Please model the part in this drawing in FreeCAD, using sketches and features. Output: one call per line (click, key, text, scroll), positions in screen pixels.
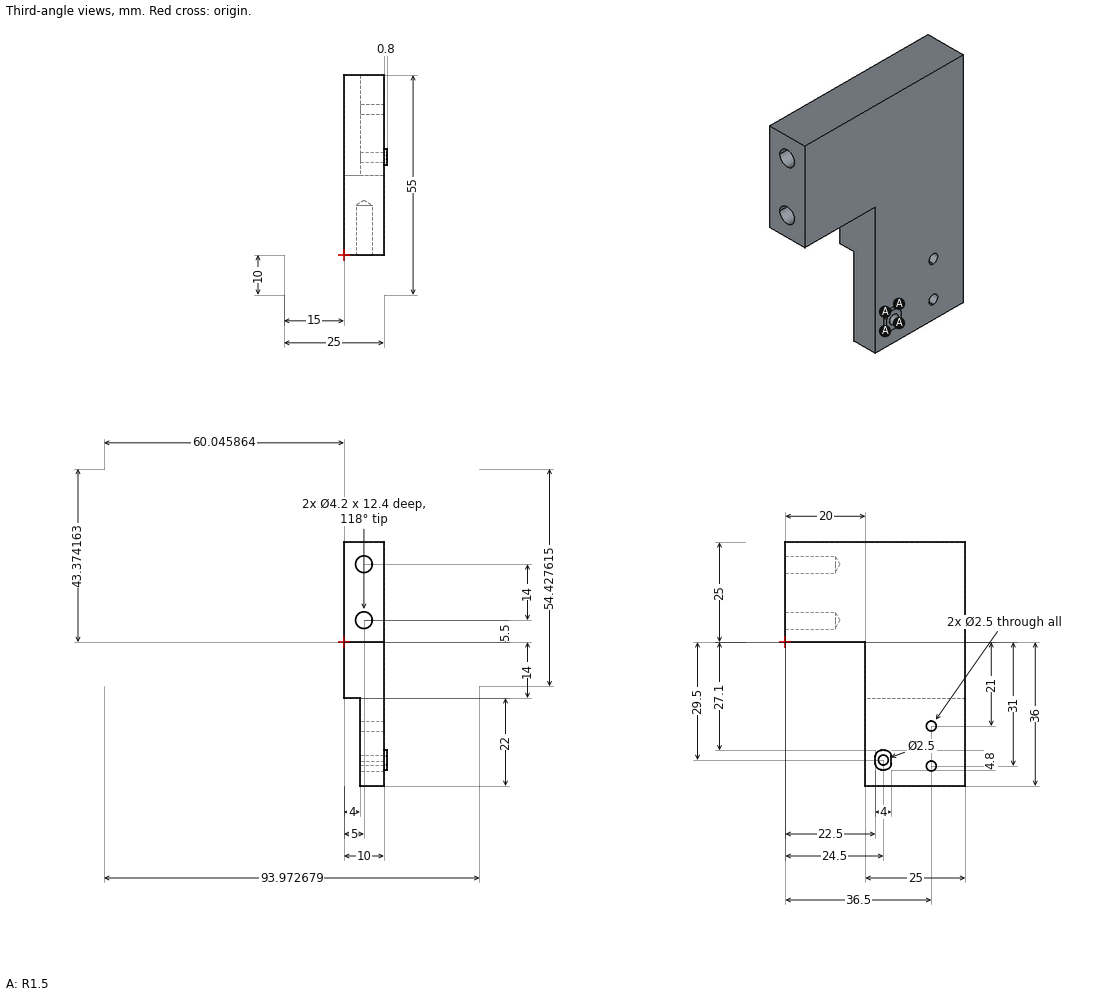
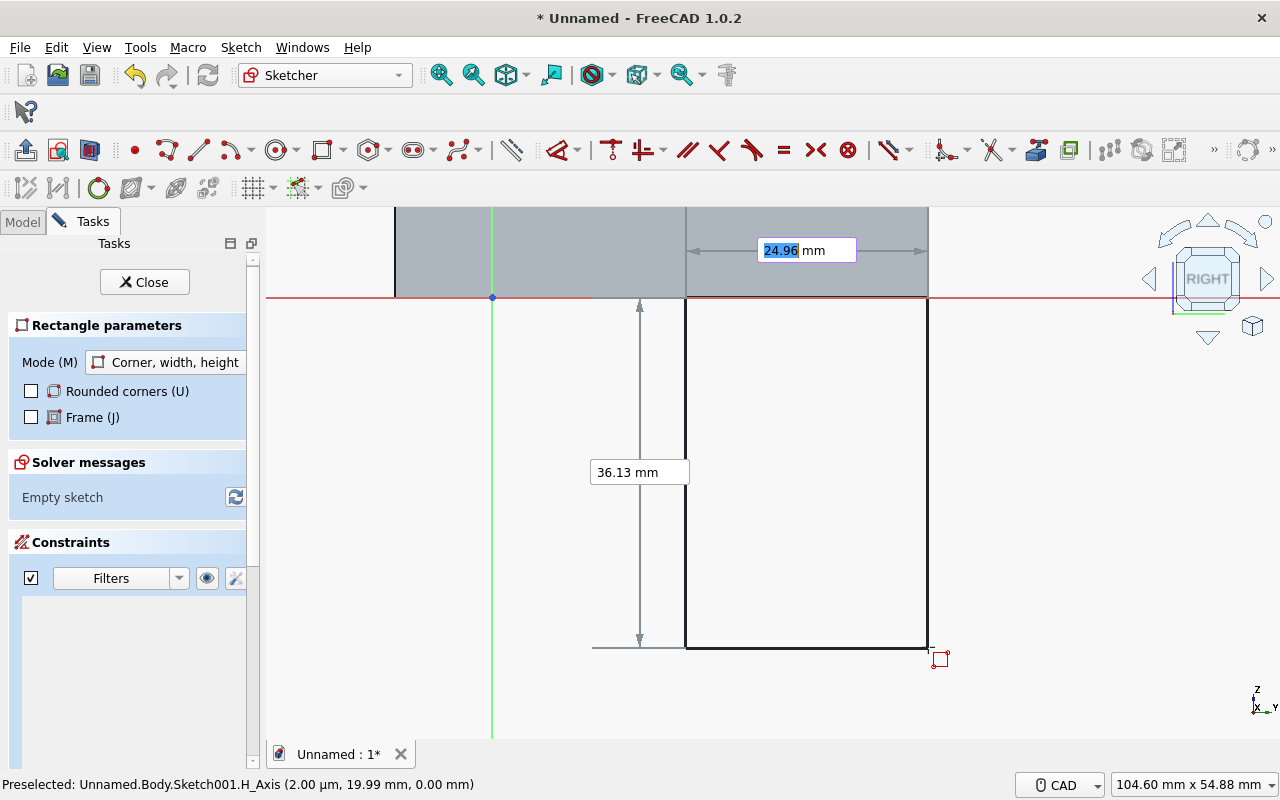
text(25)
key(Tab)
text(36)
key(Return)
key(Escape)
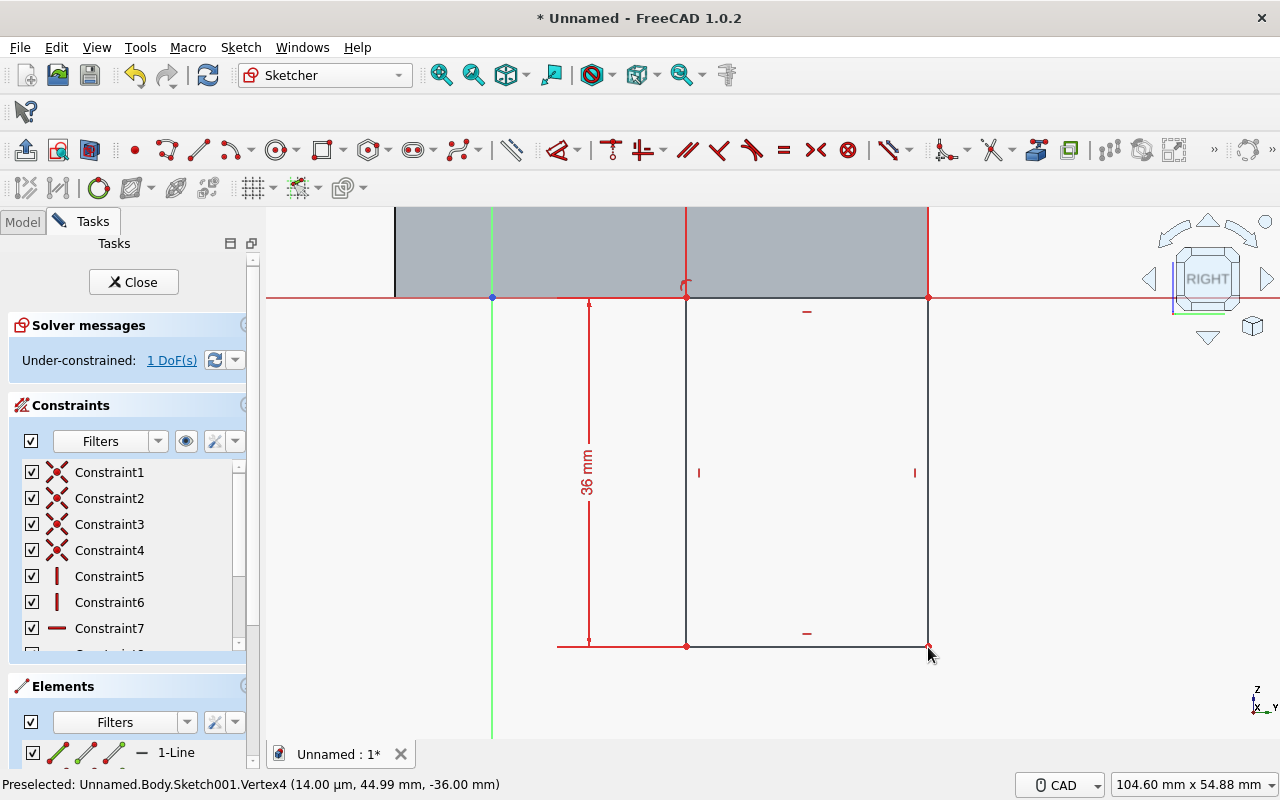
key(d)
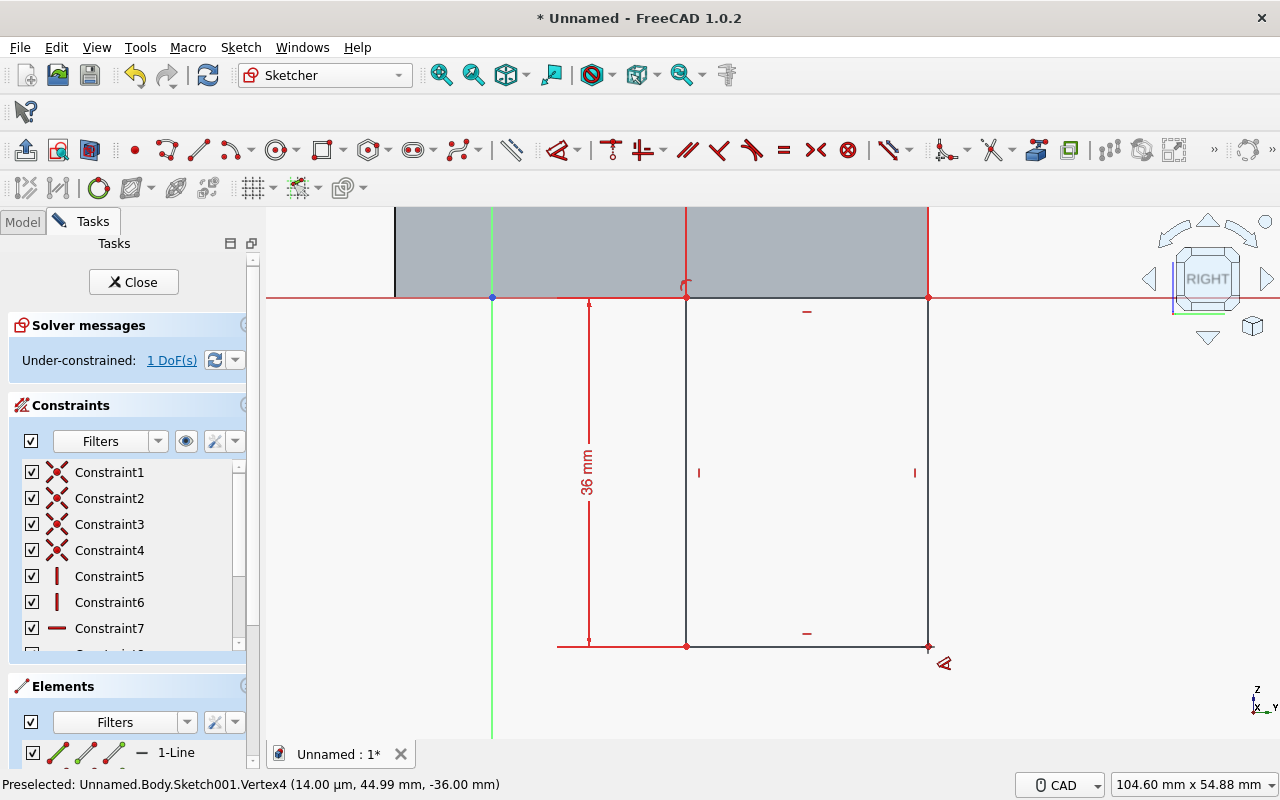
click(686, 298)
click(589, 264)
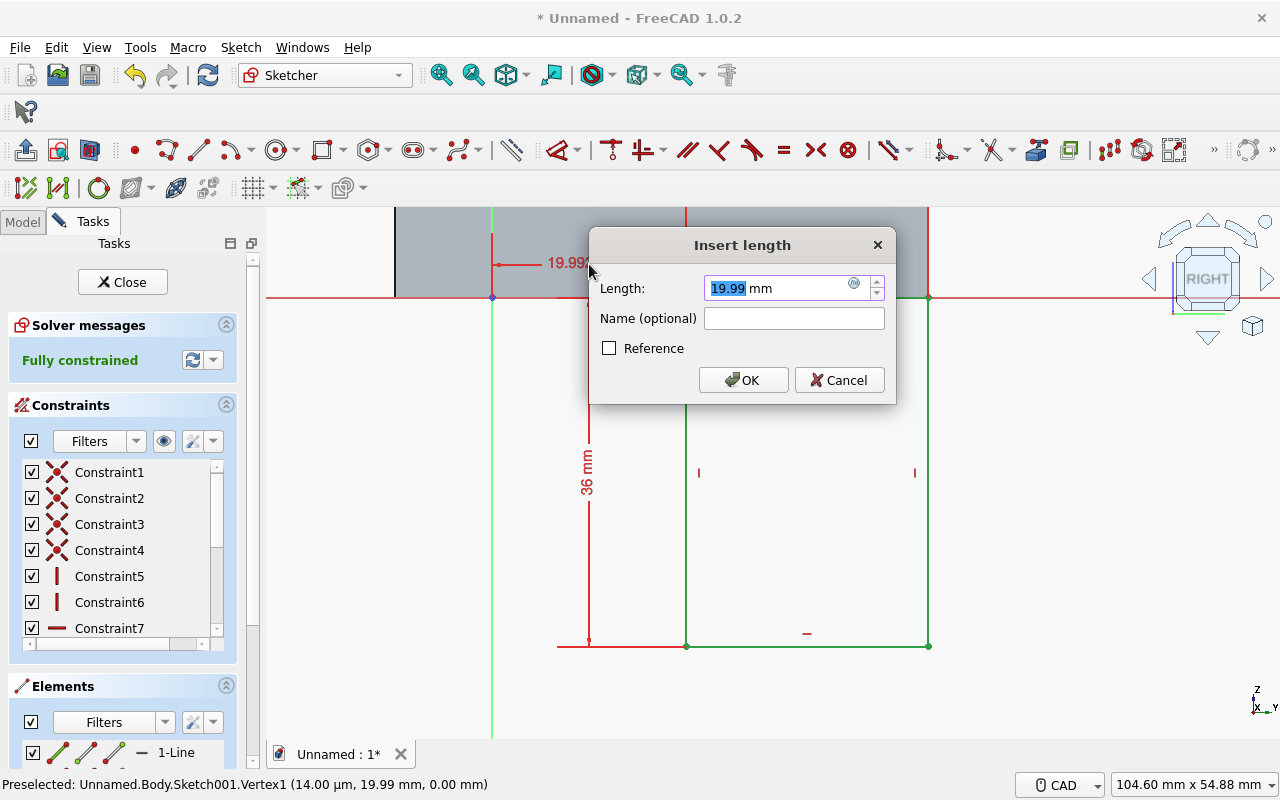
text(20)
key(Return)
key(Escape)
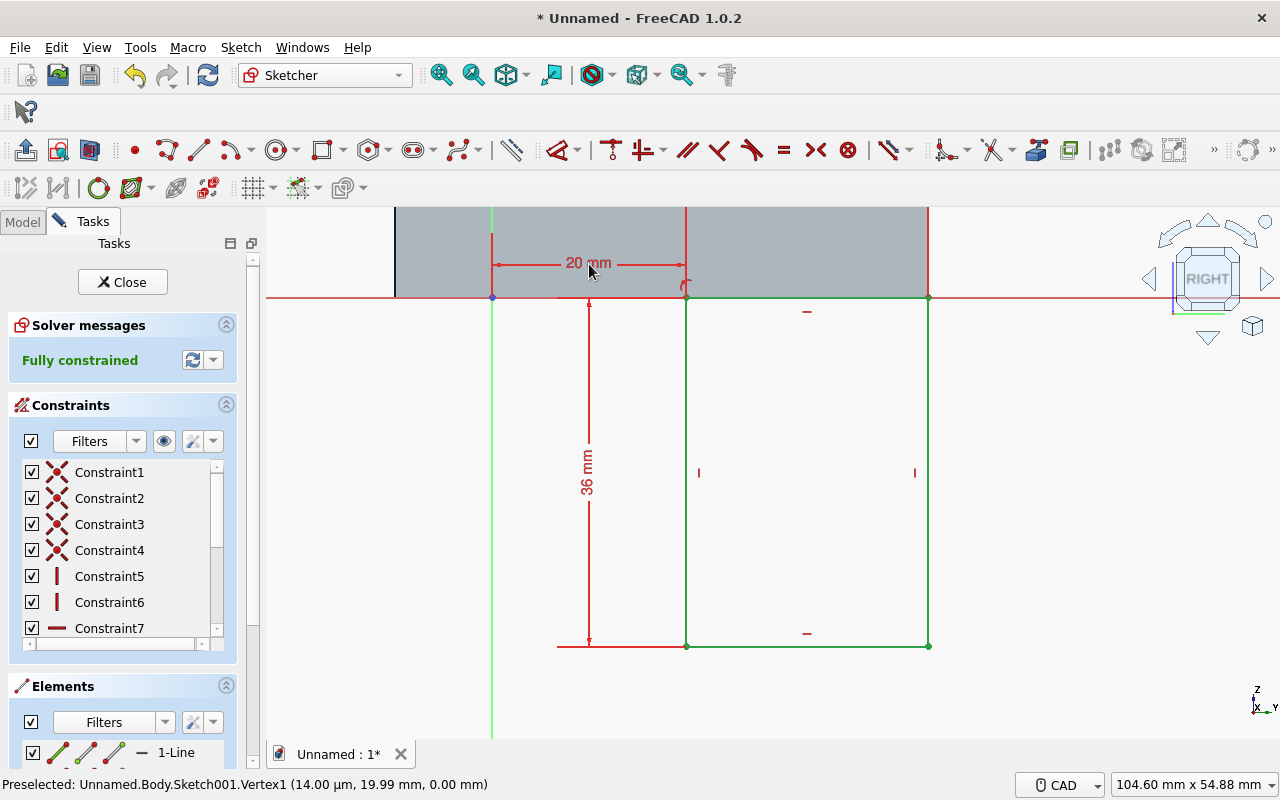
click(123, 282)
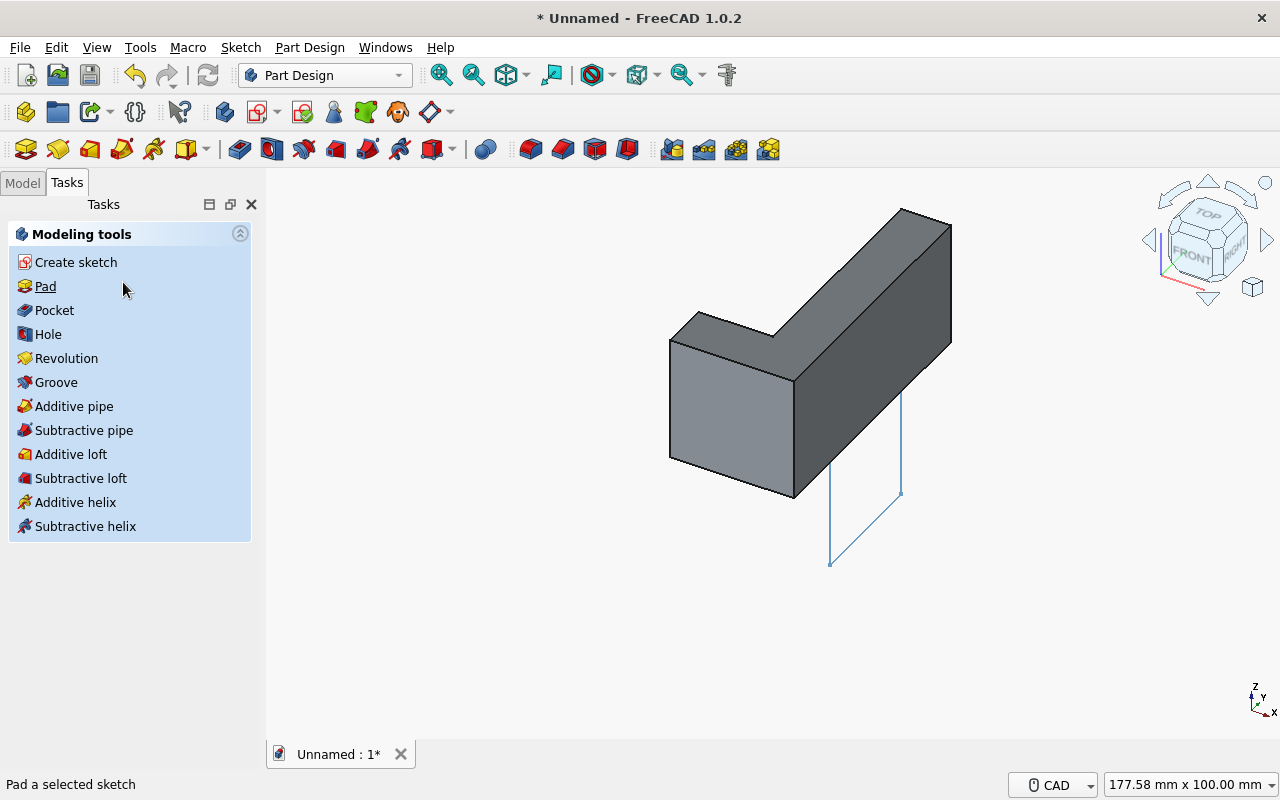
click(26, 150)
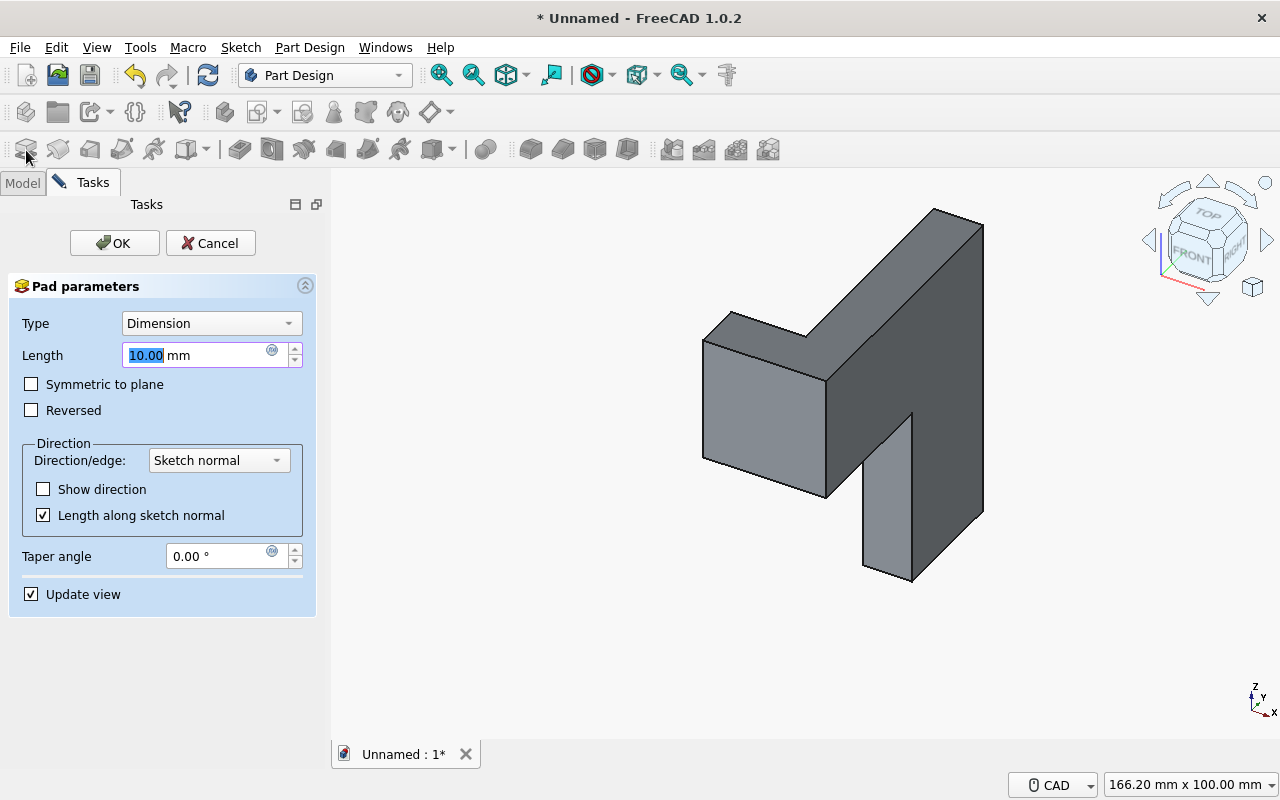
text(10)
key(Tab)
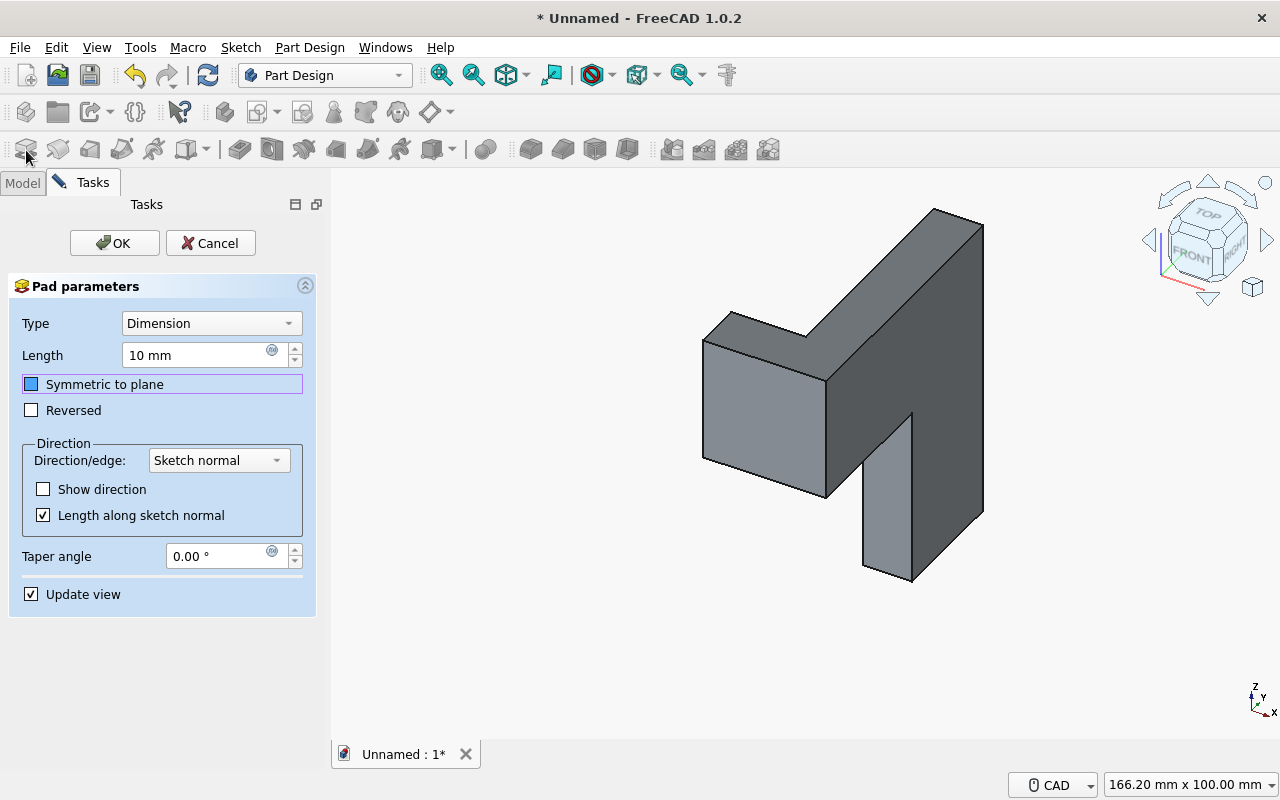
click(115, 243)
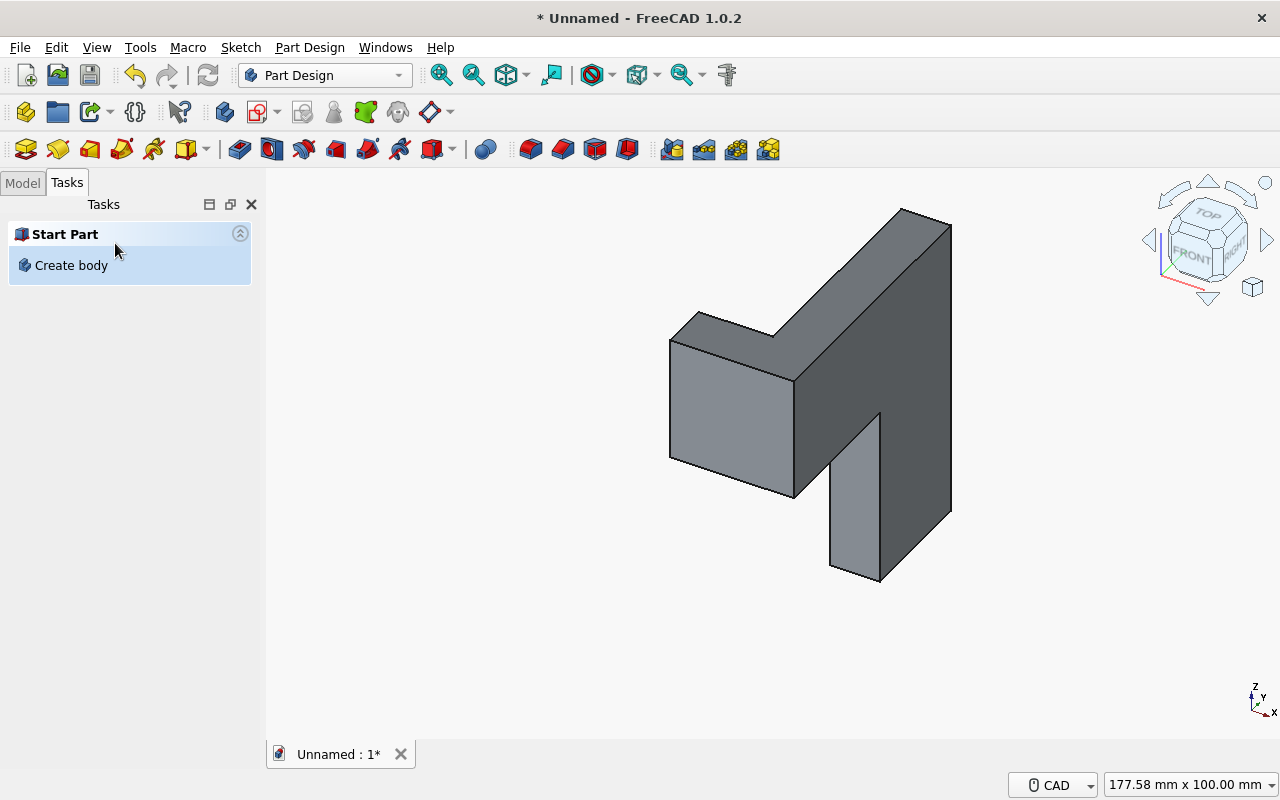
key(4)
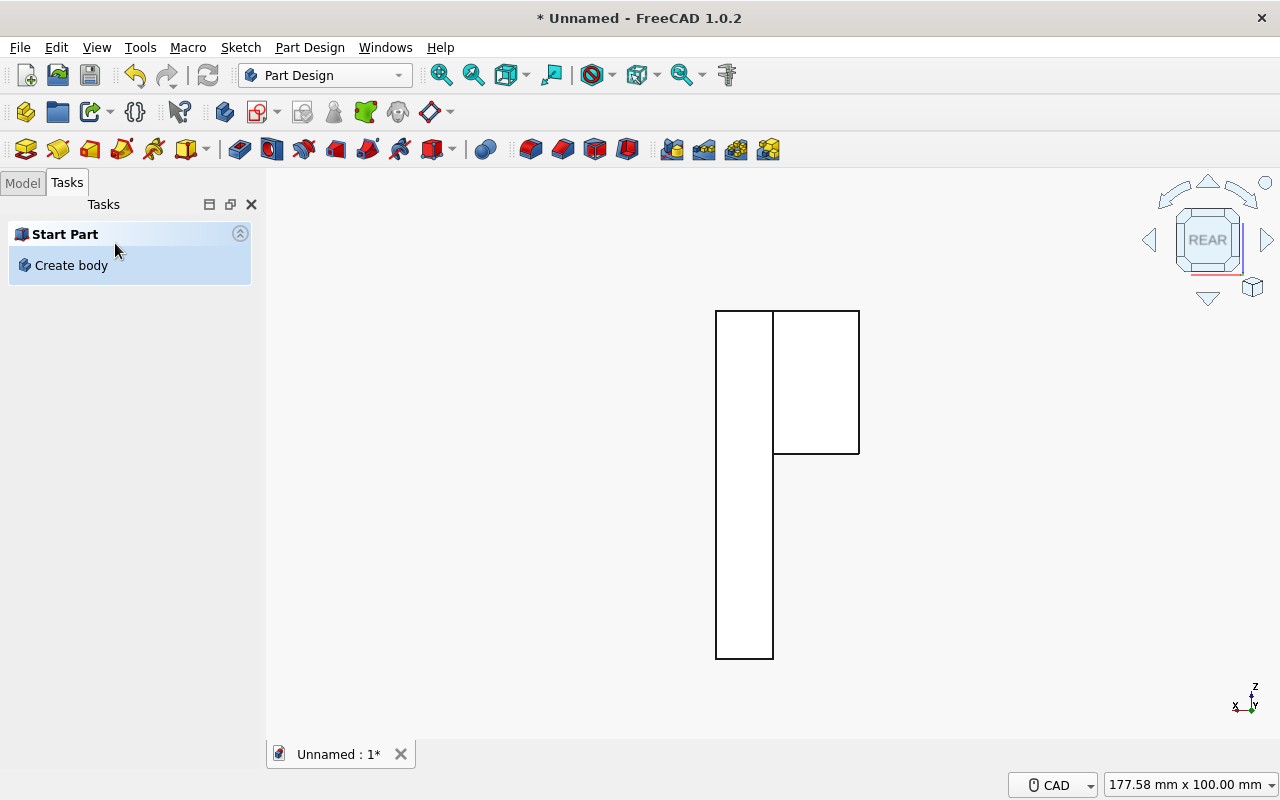
click(744, 384)